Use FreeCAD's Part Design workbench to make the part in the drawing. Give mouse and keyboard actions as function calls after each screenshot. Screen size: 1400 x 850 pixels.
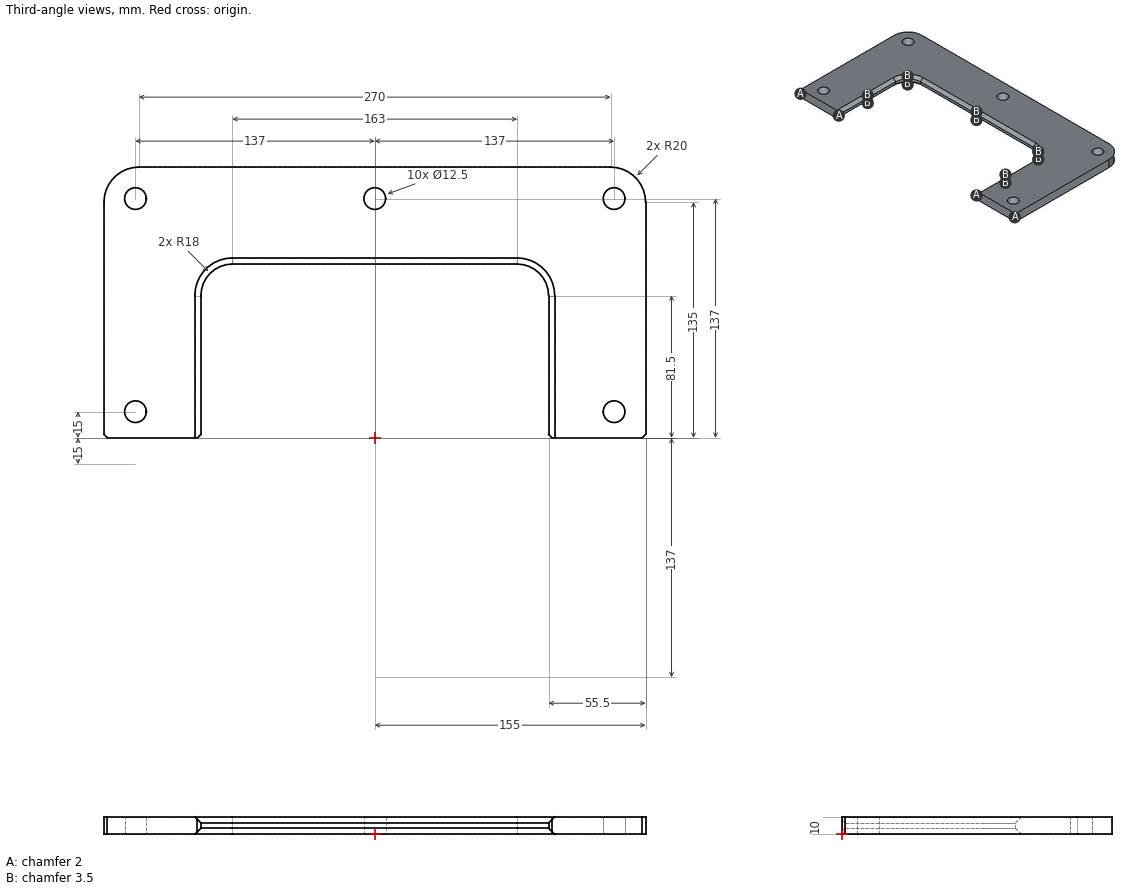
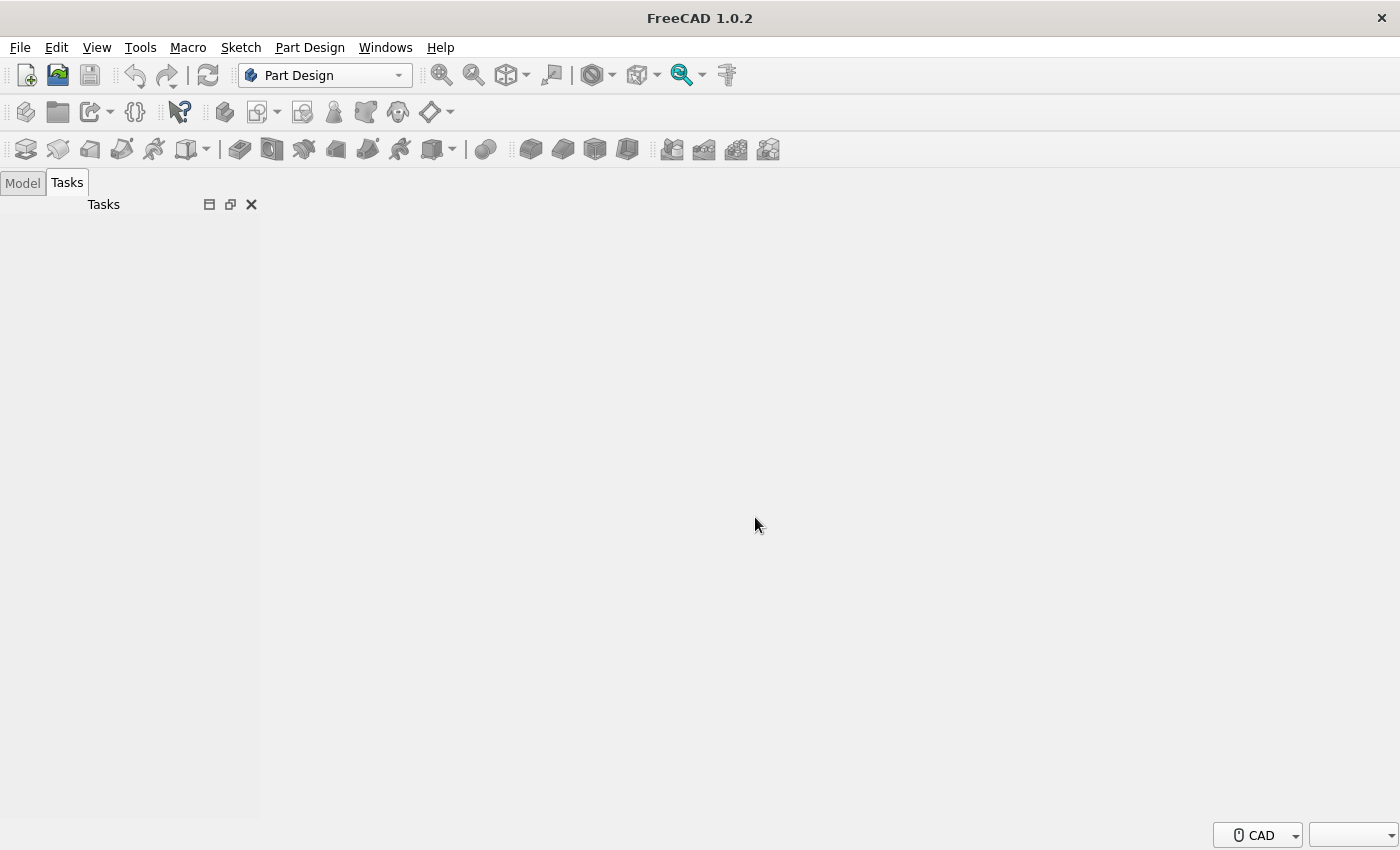
key(ctrl+n)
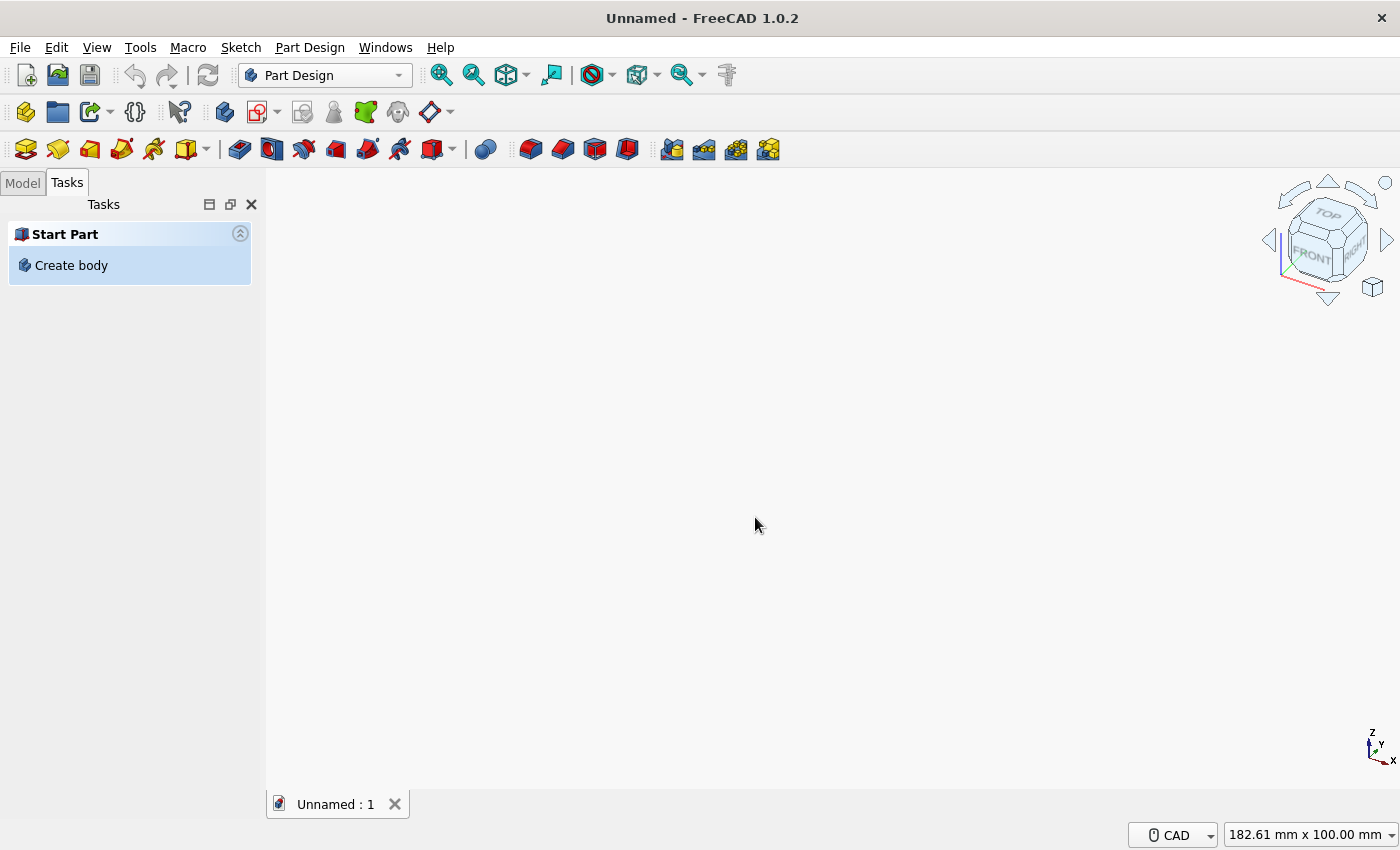
click(258, 112)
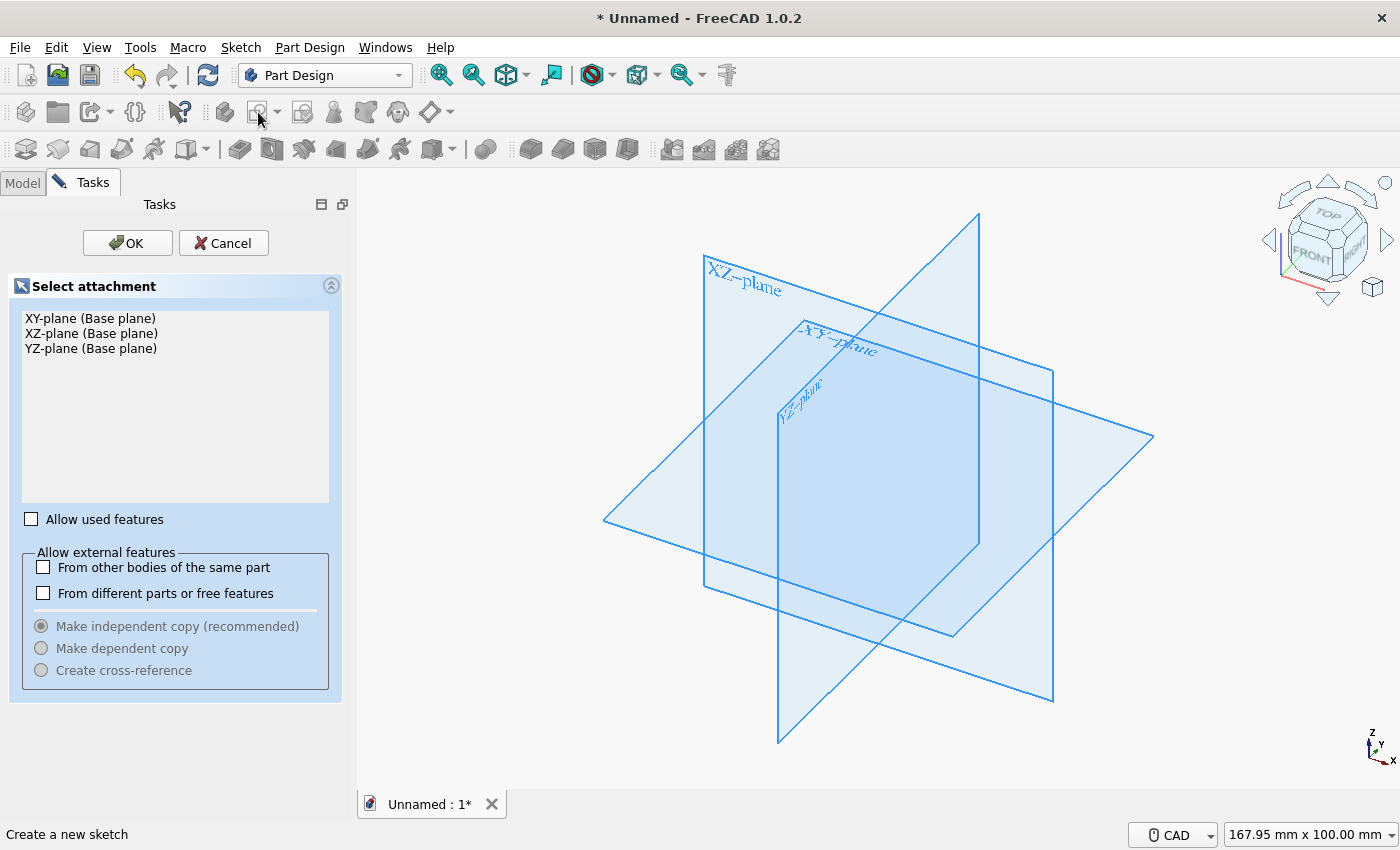
click(82, 318)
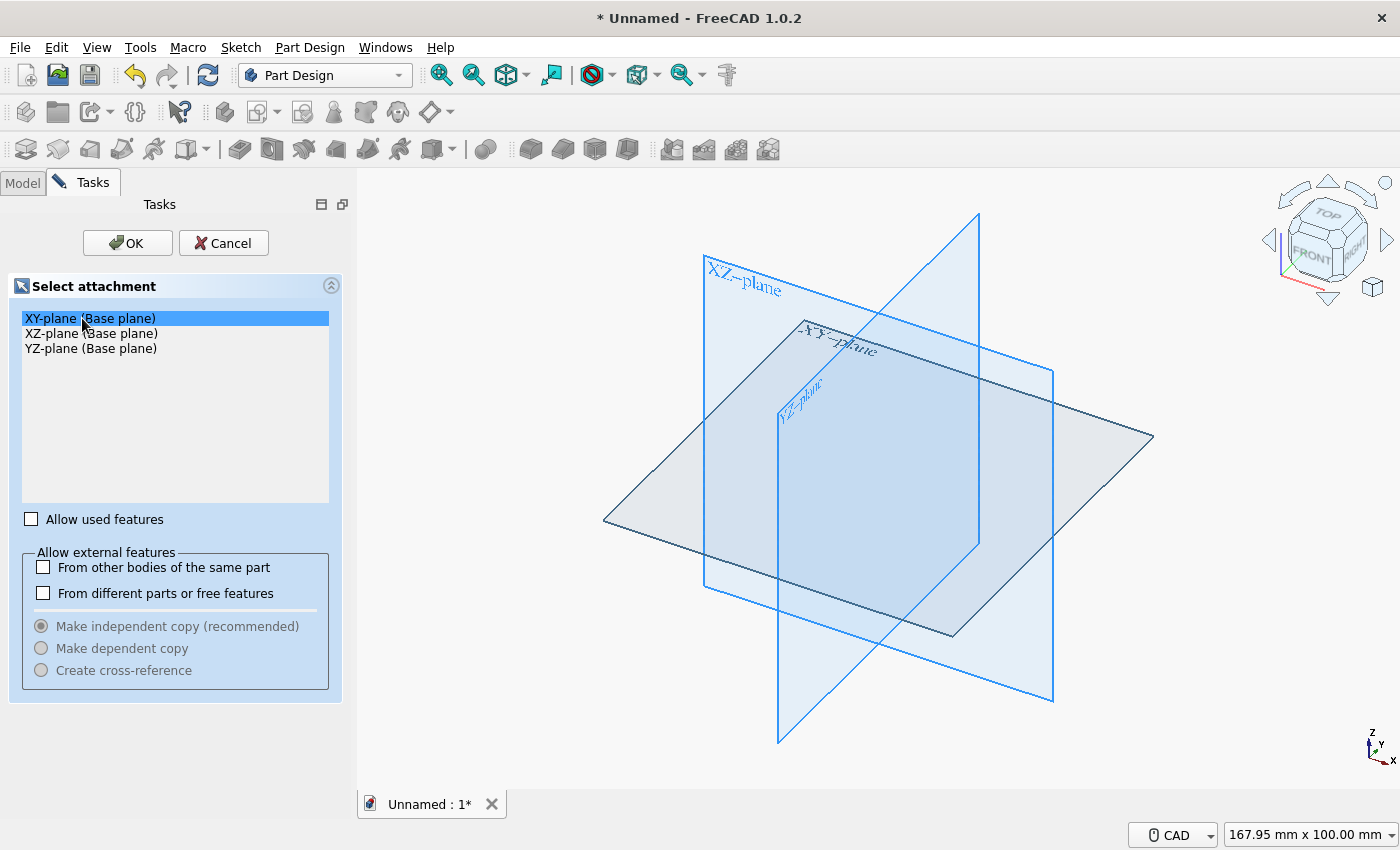
click(128, 243)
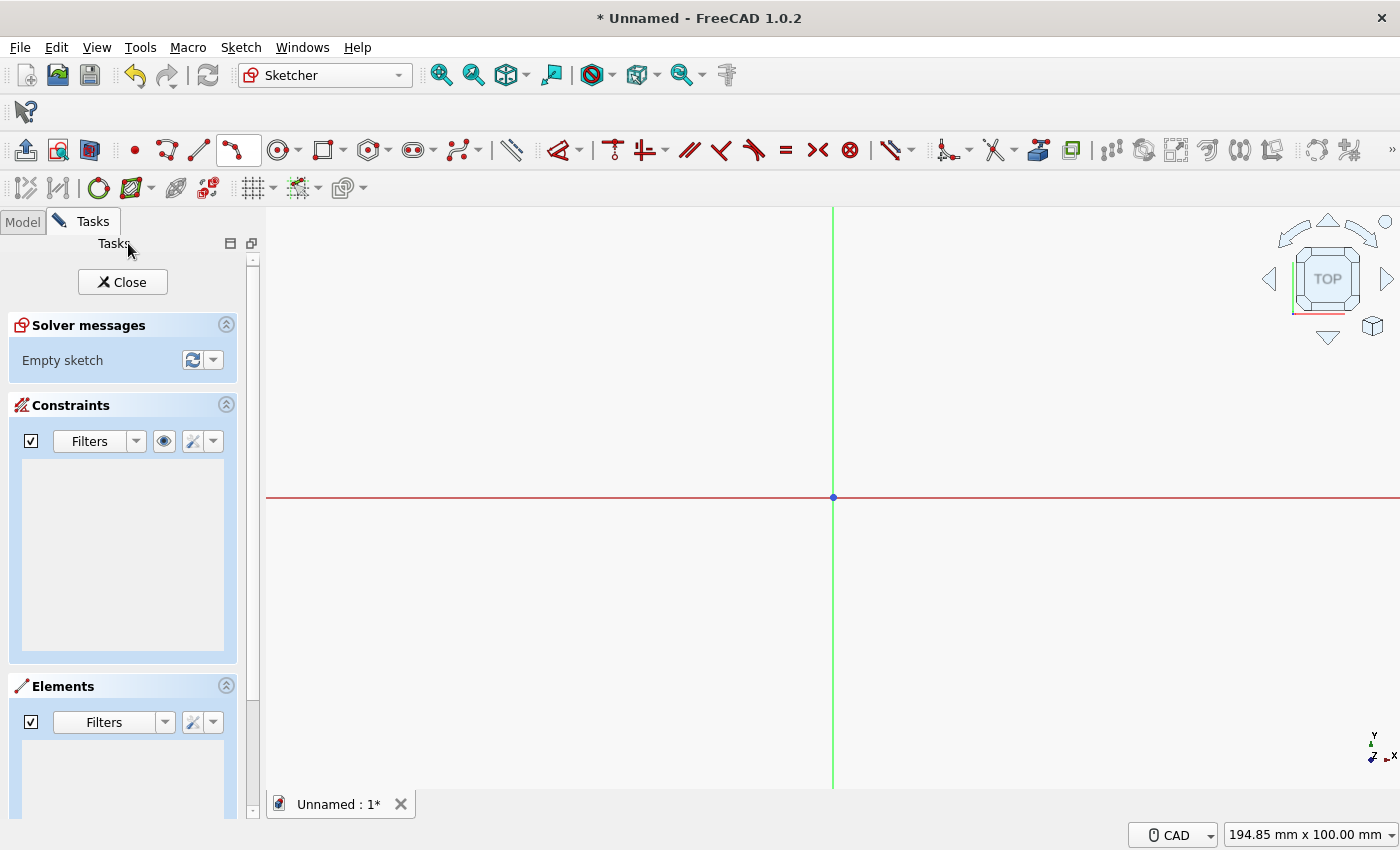
scroll(725, 761, down, 5)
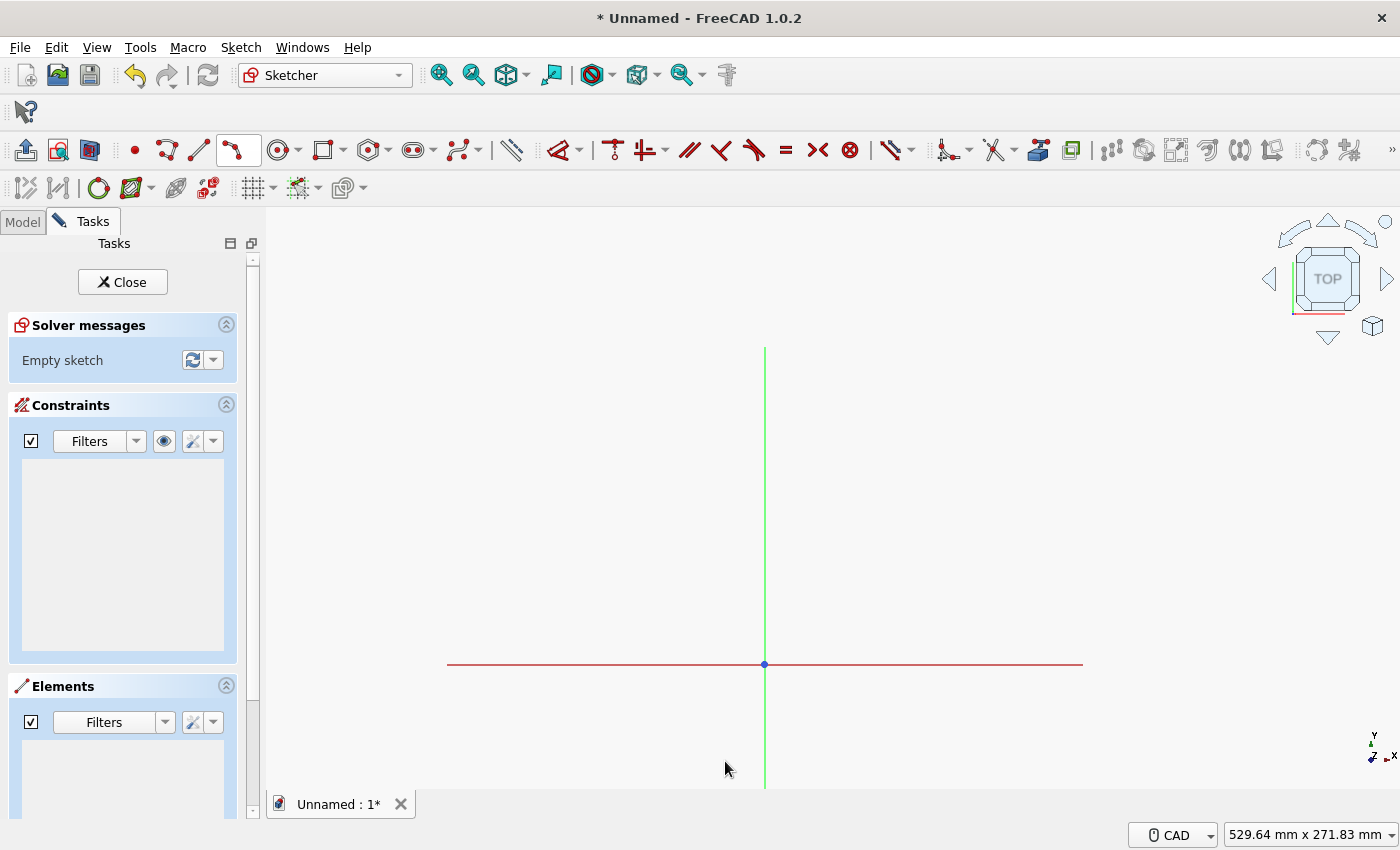
key(g)
key(l)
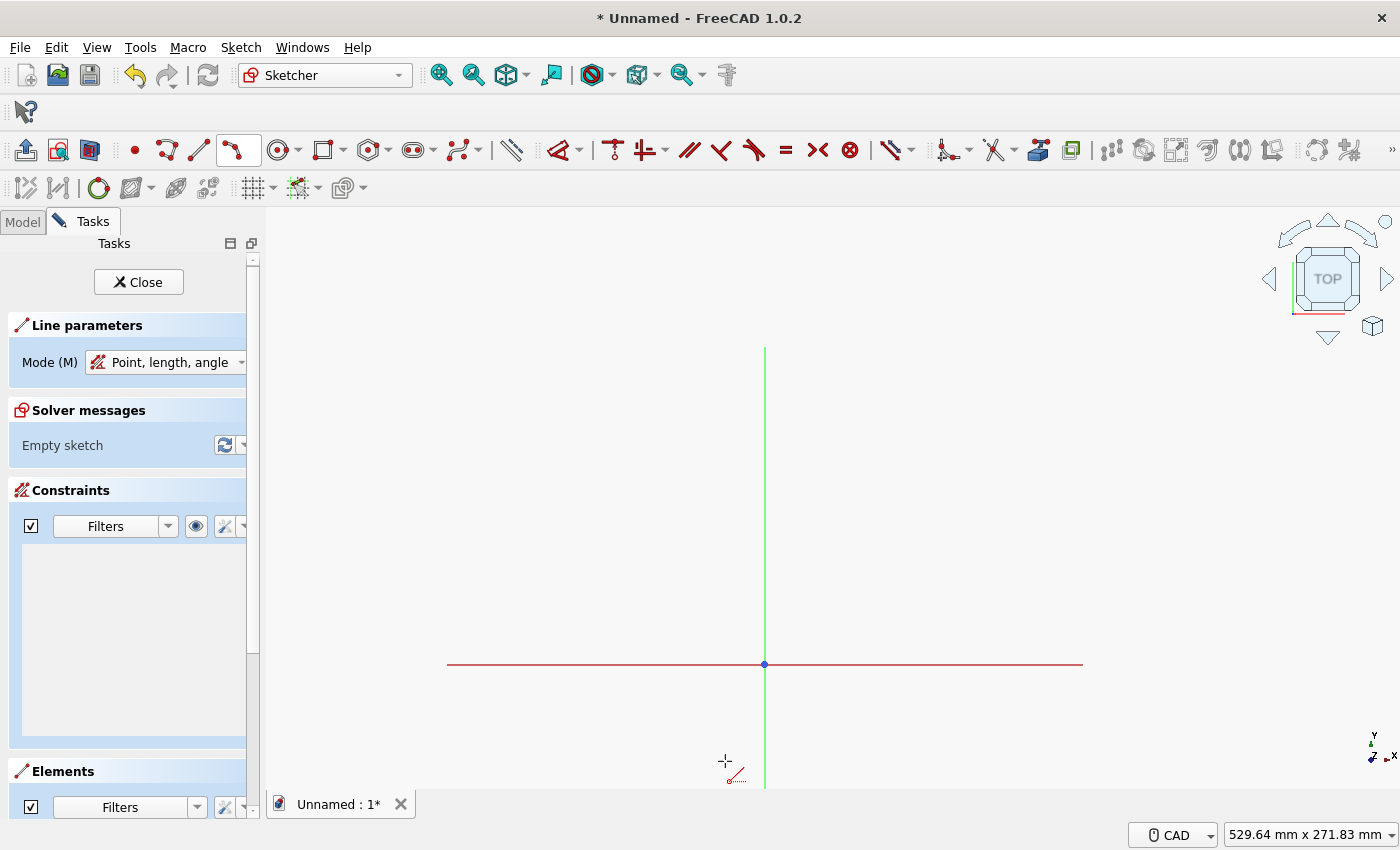
click(590, 452)
click(939, 452)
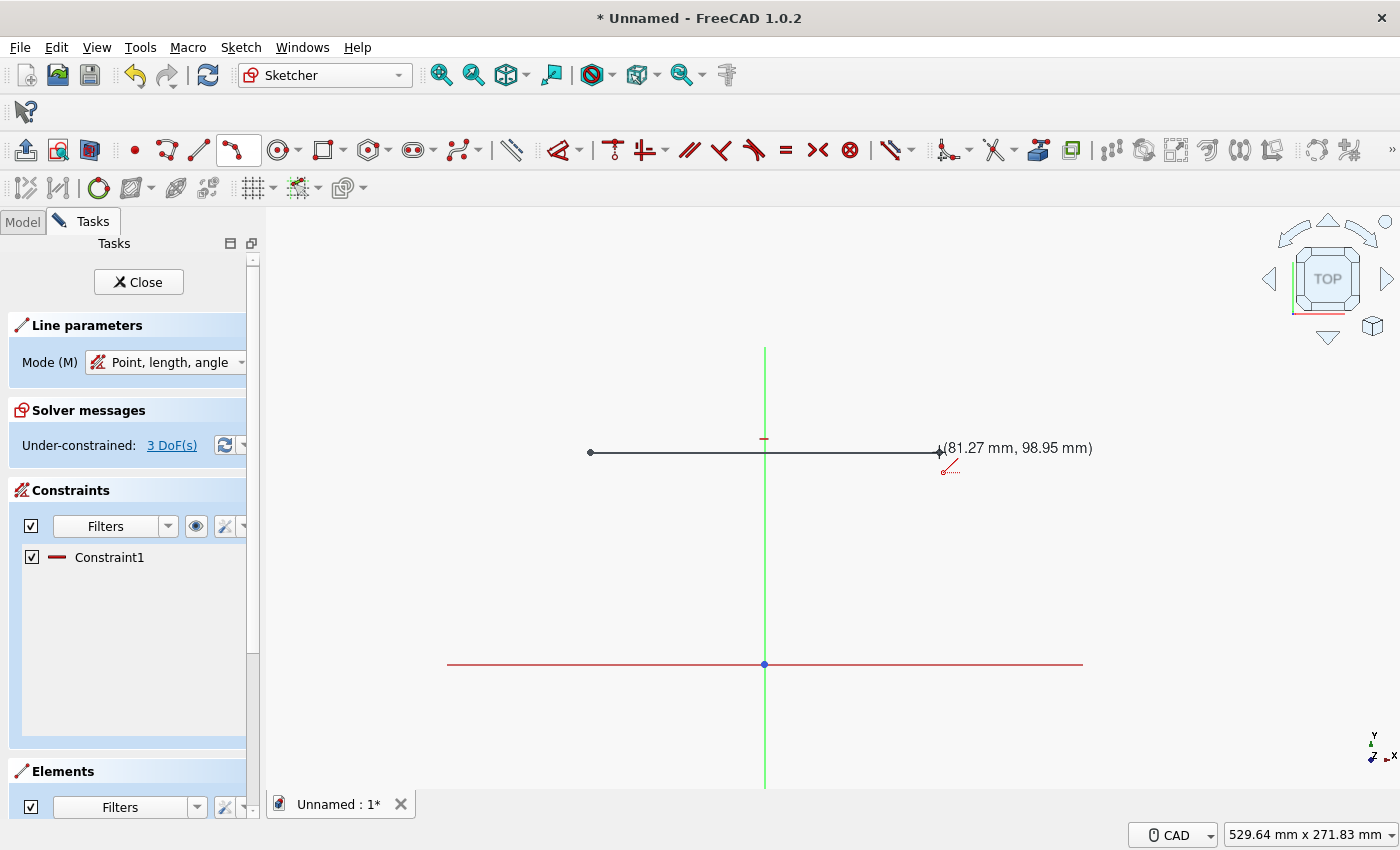
key(g)
key(m)